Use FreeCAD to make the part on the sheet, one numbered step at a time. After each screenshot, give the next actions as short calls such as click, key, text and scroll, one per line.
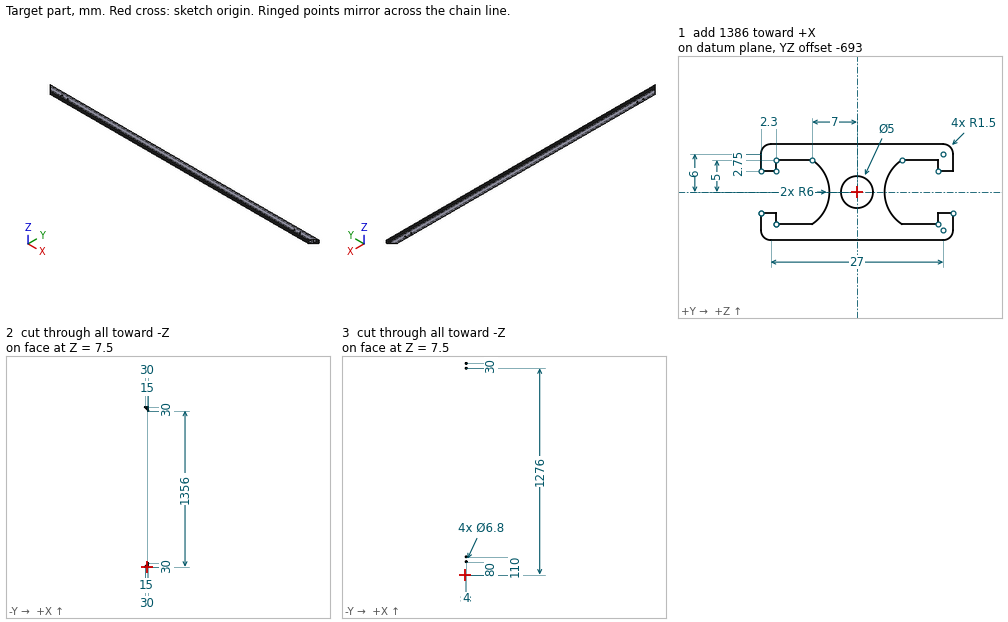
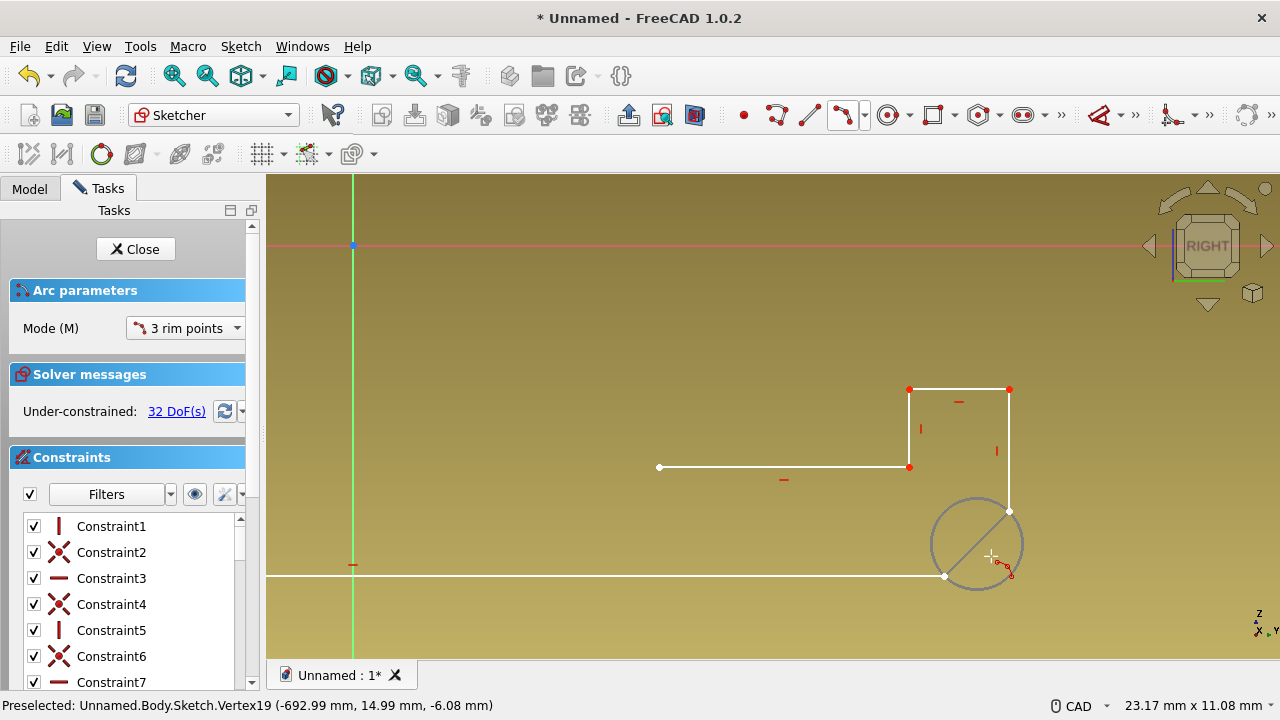
click(990, 555)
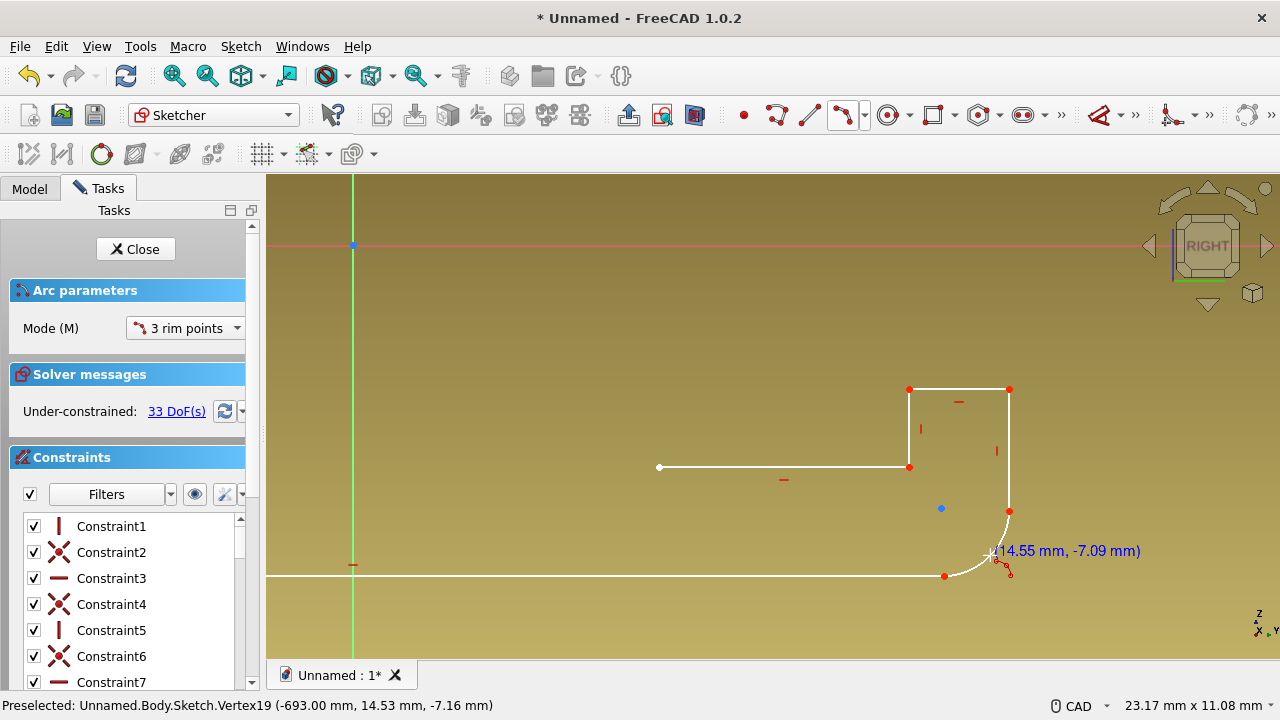
click(660, 467)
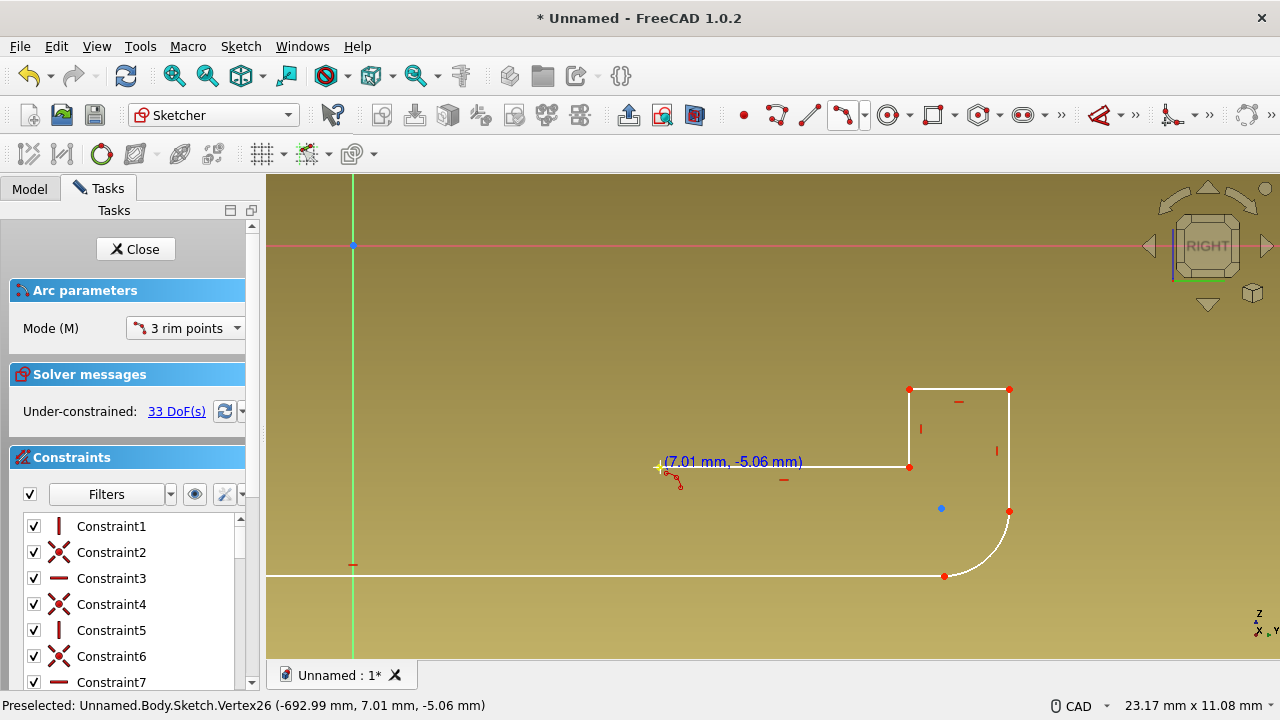
scroll(991, 556, down, 4)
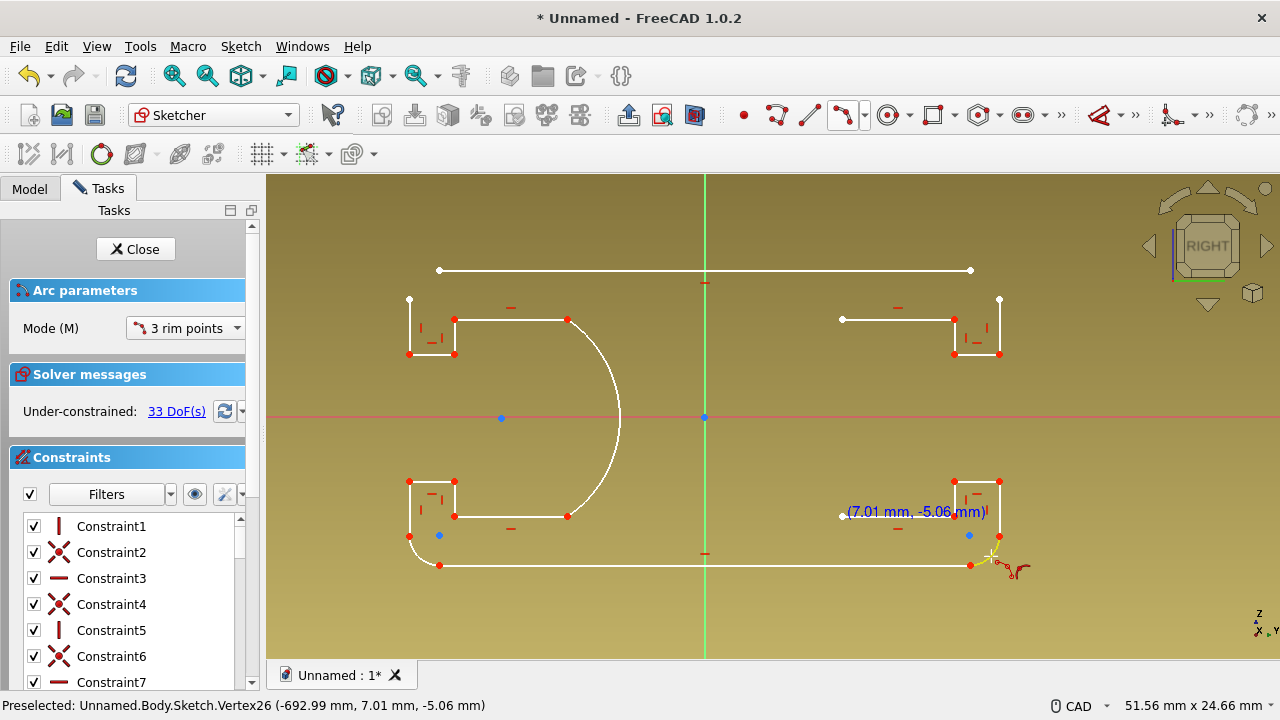
click(843, 320)
click(792, 394)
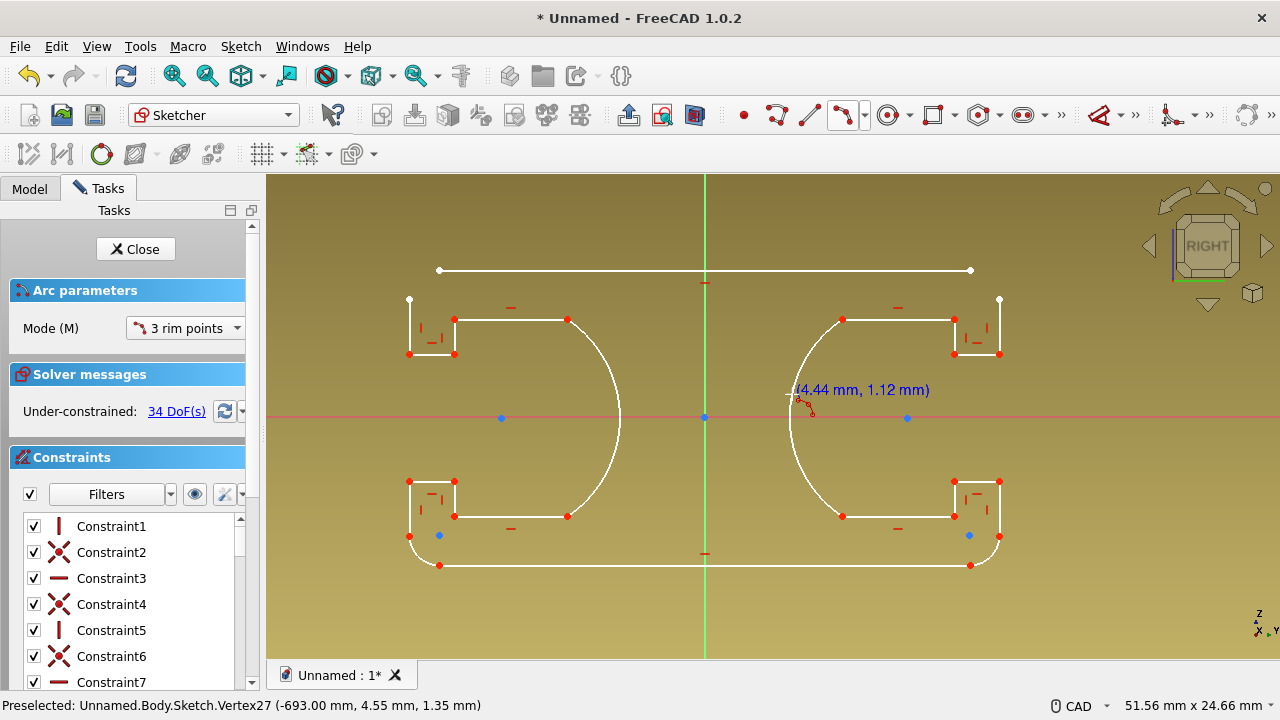
click(1000, 300)
click(971, 271)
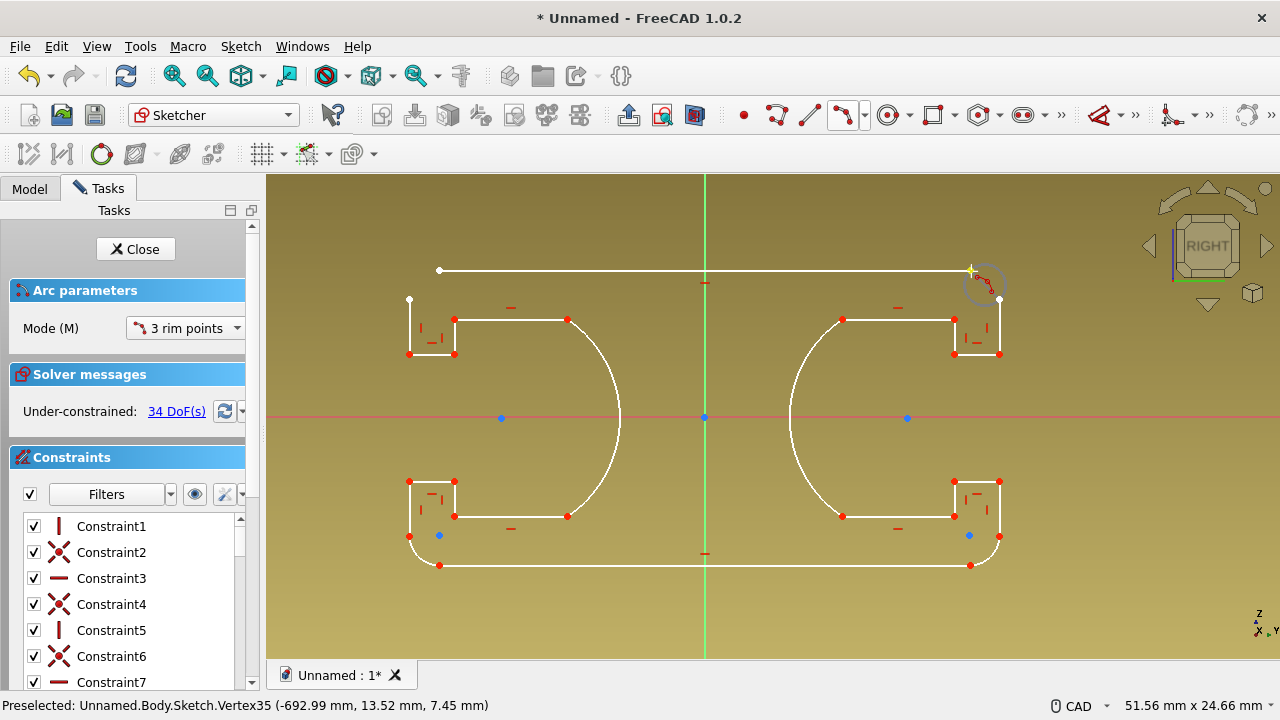
scroll(991, 278, up, 4)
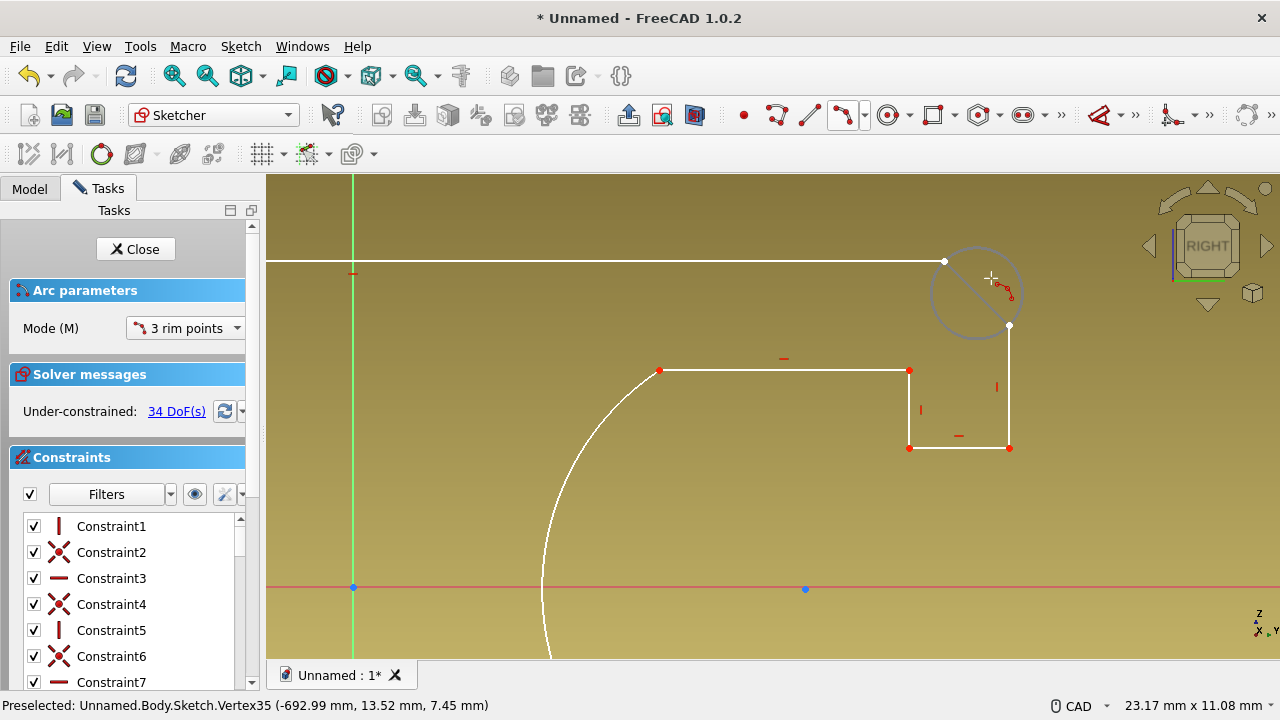
click(990, 278)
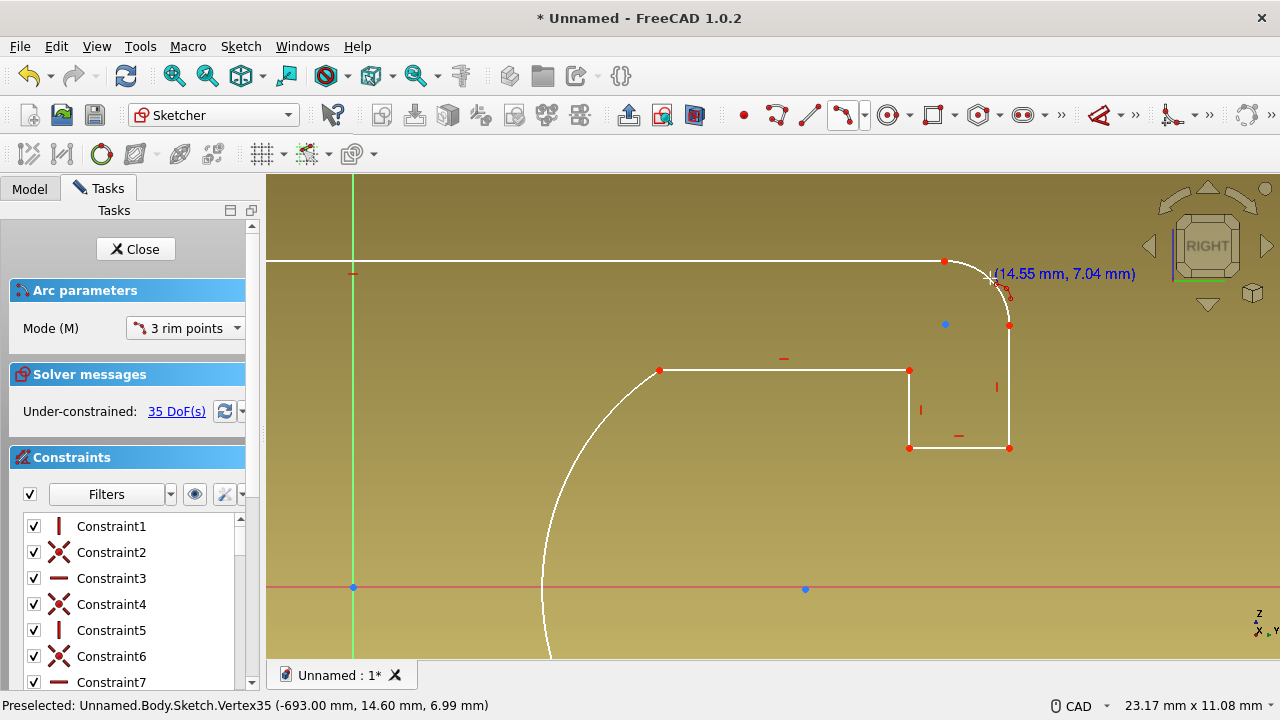
scroll(991, 277, down, 4)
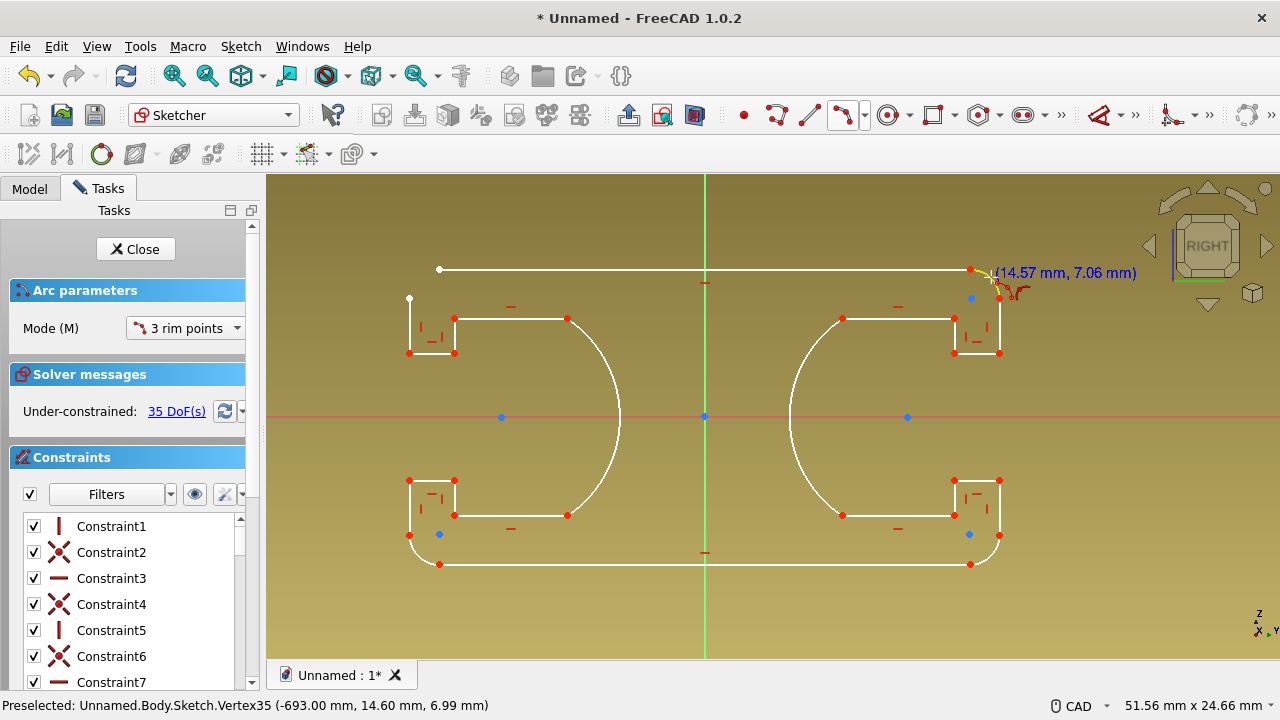
click(440, 270)
click(410, 299)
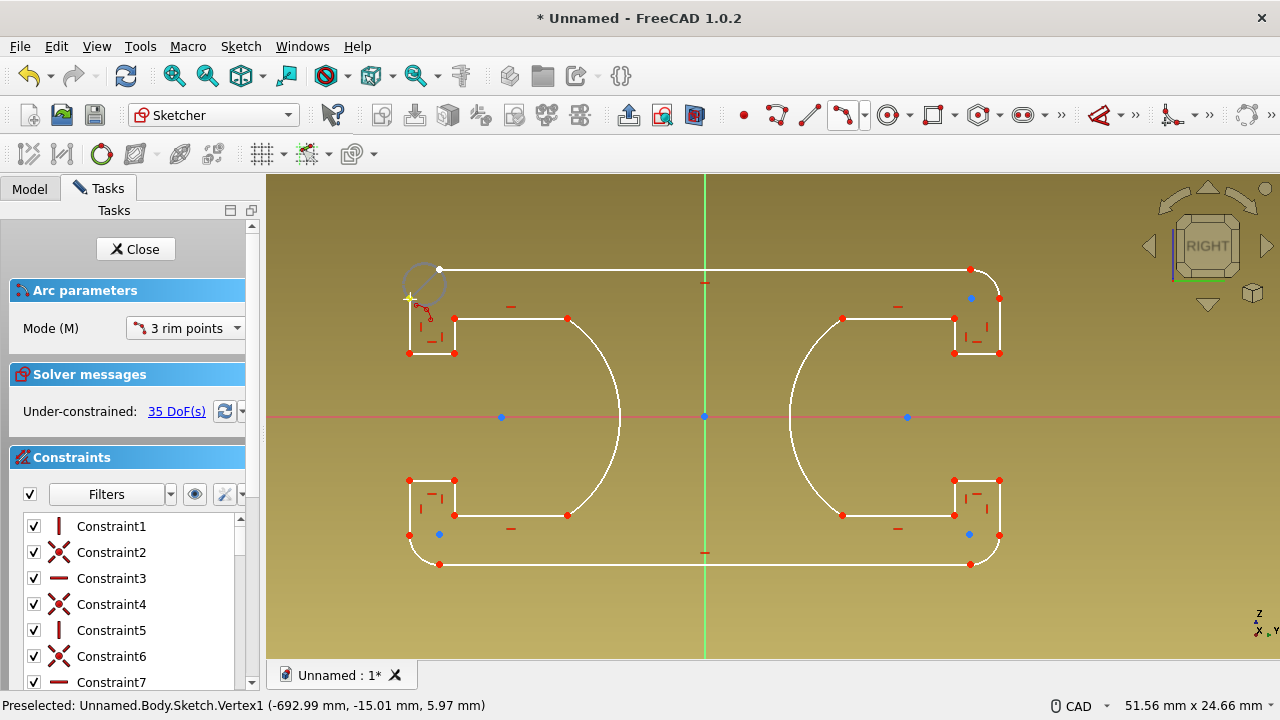
scroll(418, 278, up, 4)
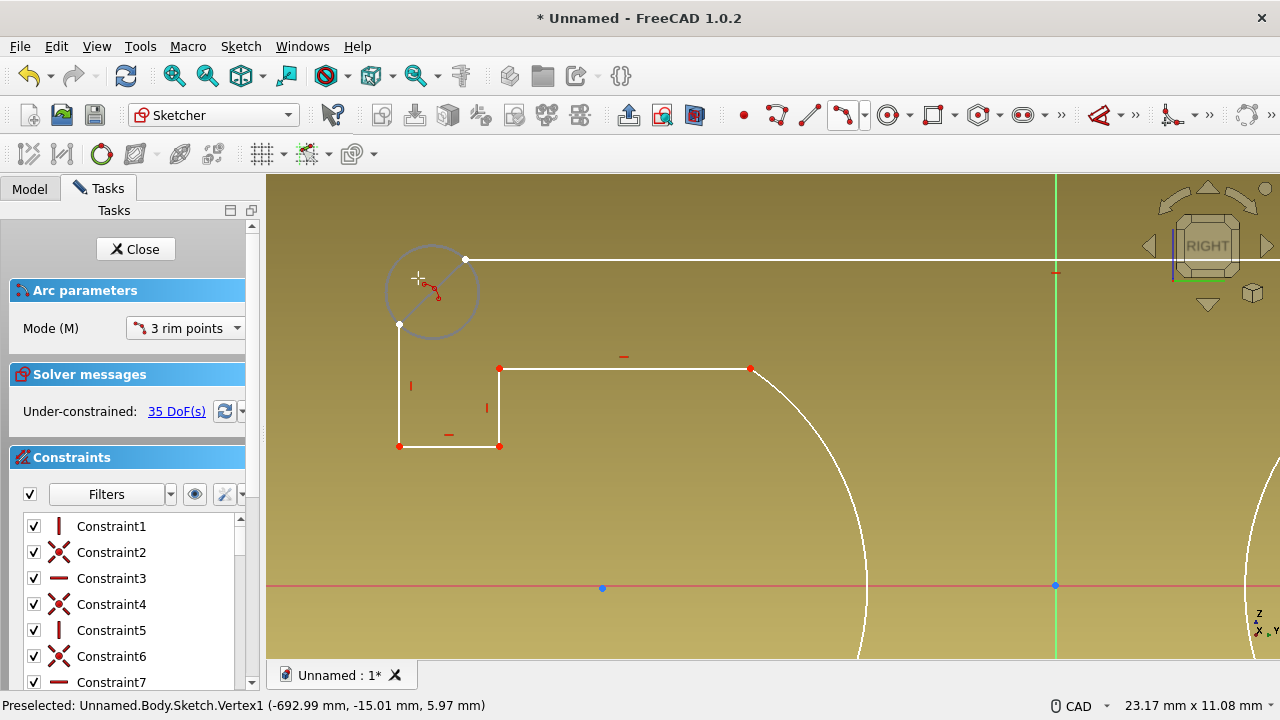
click(419, 277)